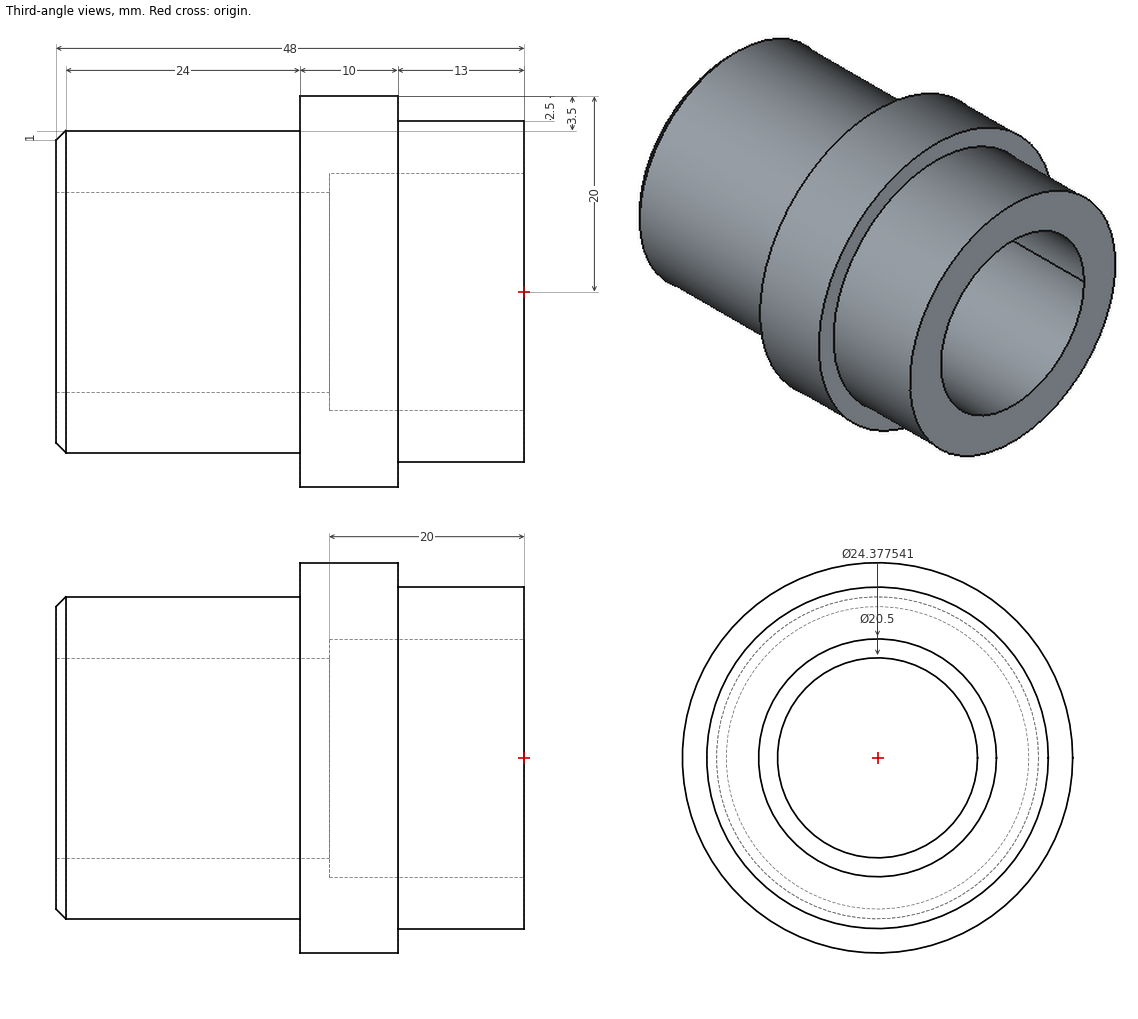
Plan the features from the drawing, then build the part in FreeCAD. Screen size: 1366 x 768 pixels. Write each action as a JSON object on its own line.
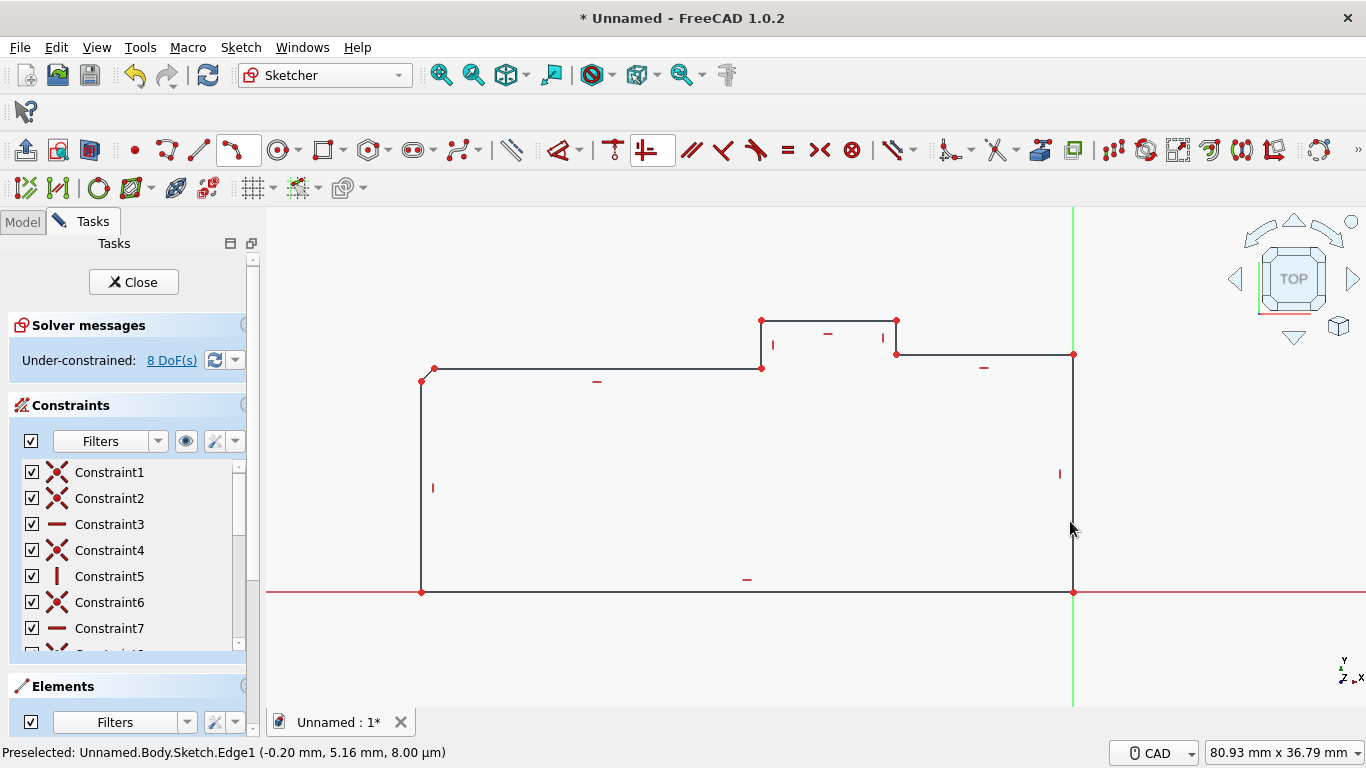
{"action": "left_click", "coordinate": [558, 150]}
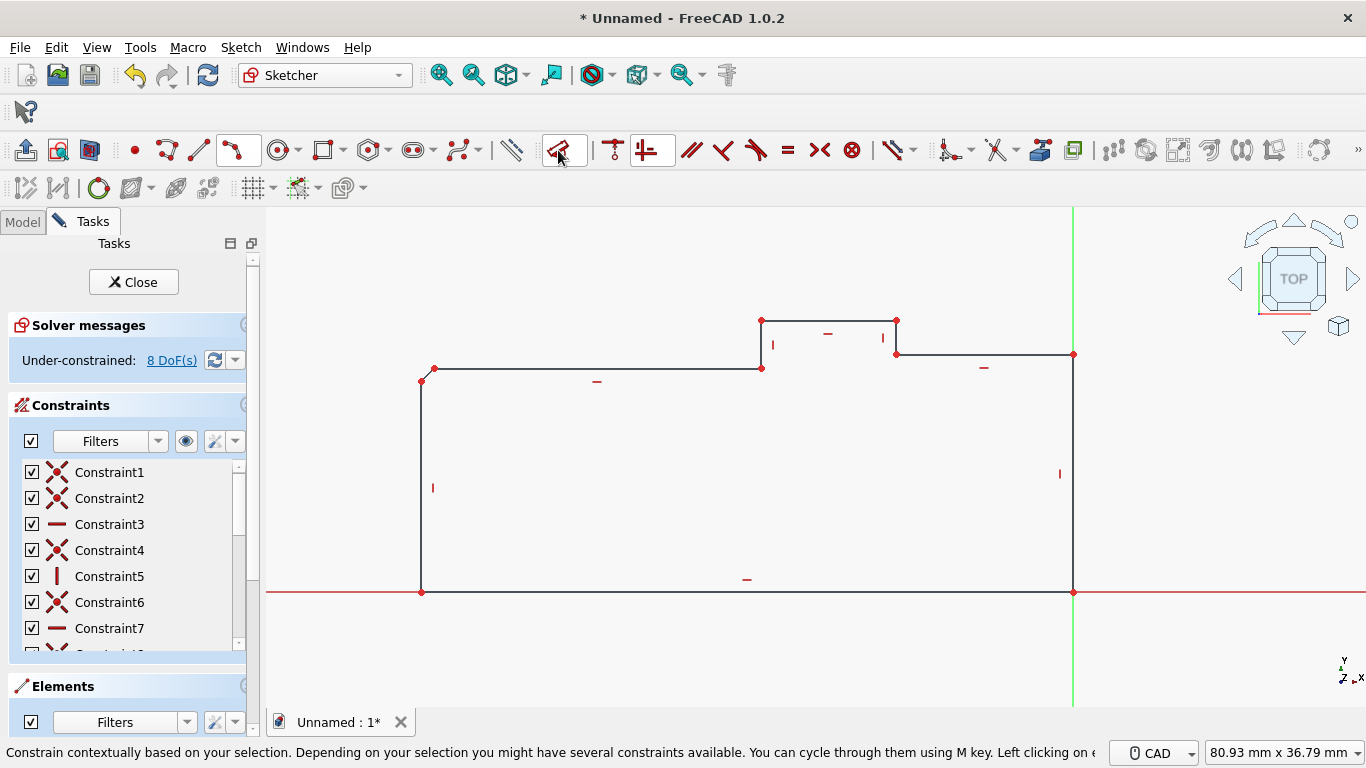
{"action": "left_click", "coordinate": [1020, 355]}
{"action": "left_click", "coordinate": [985, 321]}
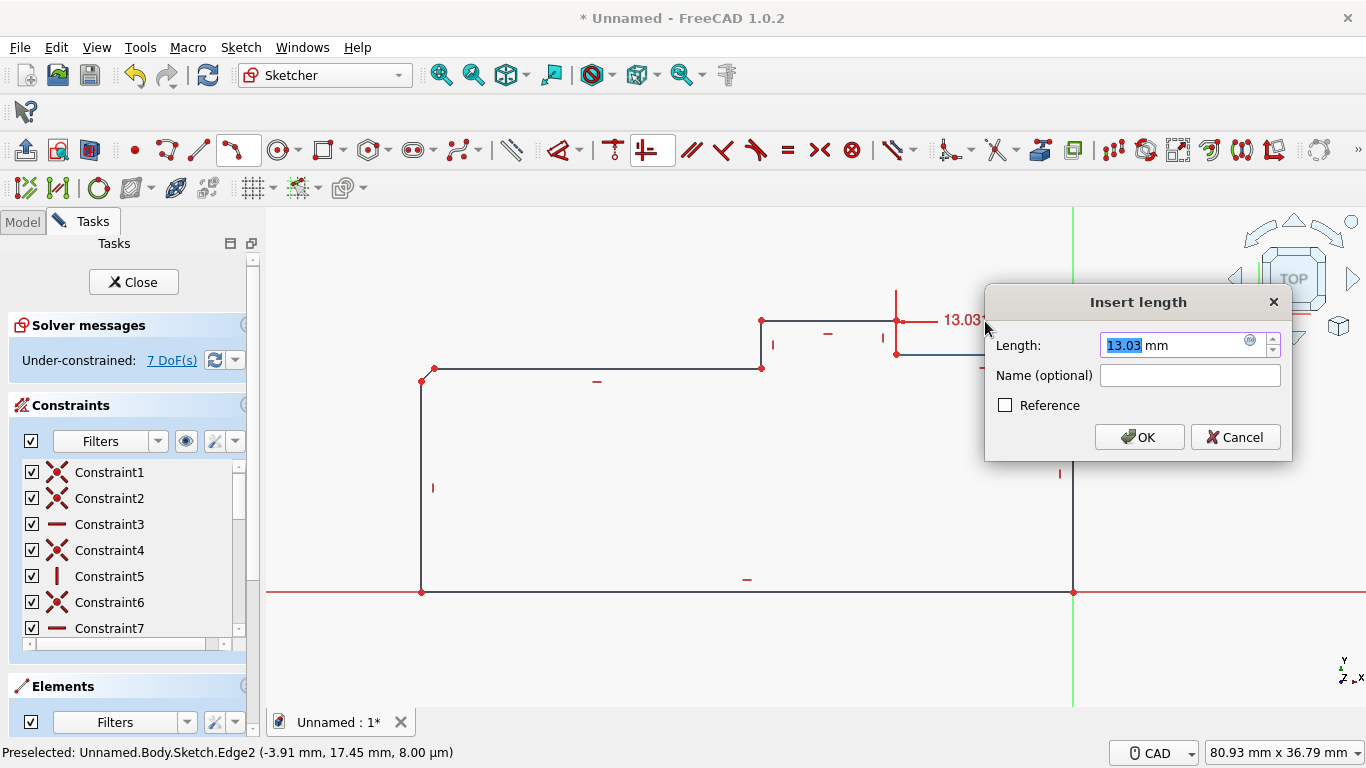
{"action": "type", "text": "13"}
{"action": "key", "text": "Return"}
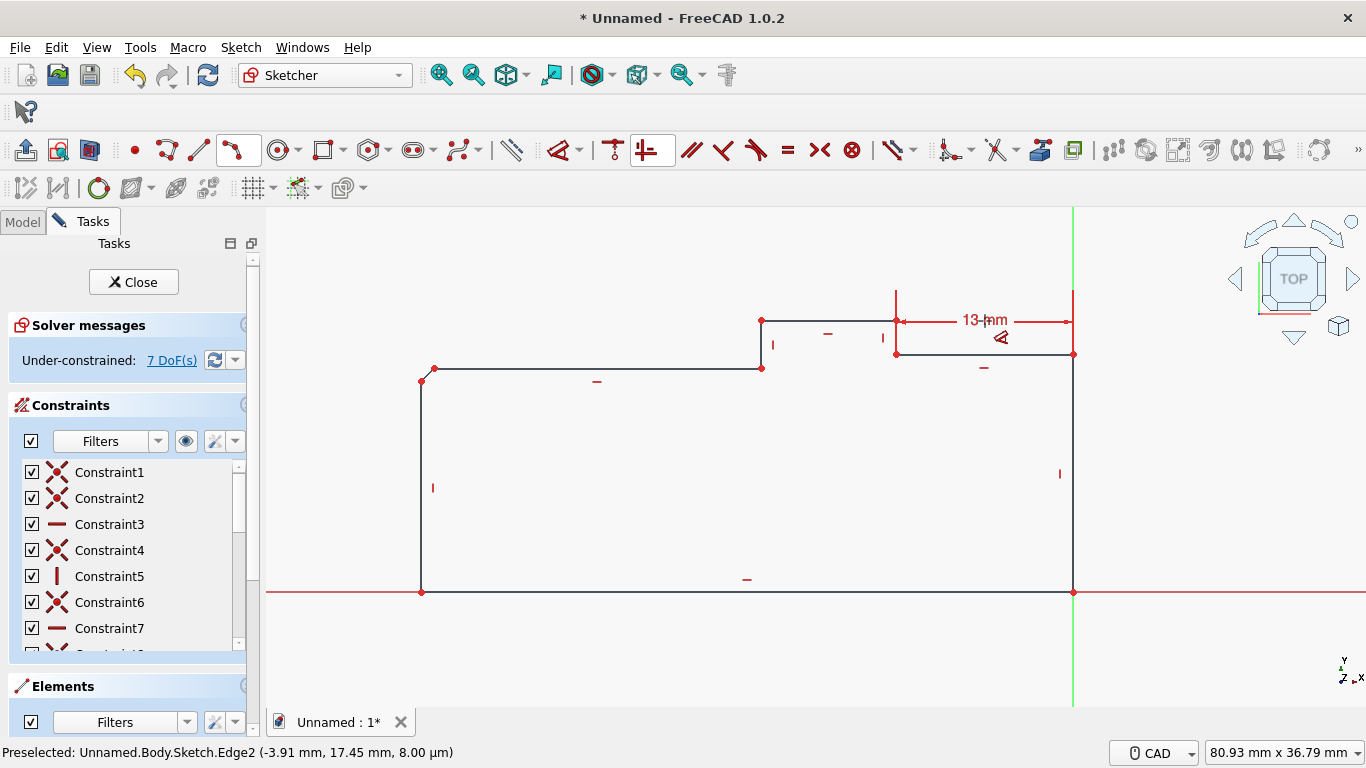
{"action": "left_click", "coordinate": [856, 321]}
{"action": "left_click", "coordinate": [829, 287]}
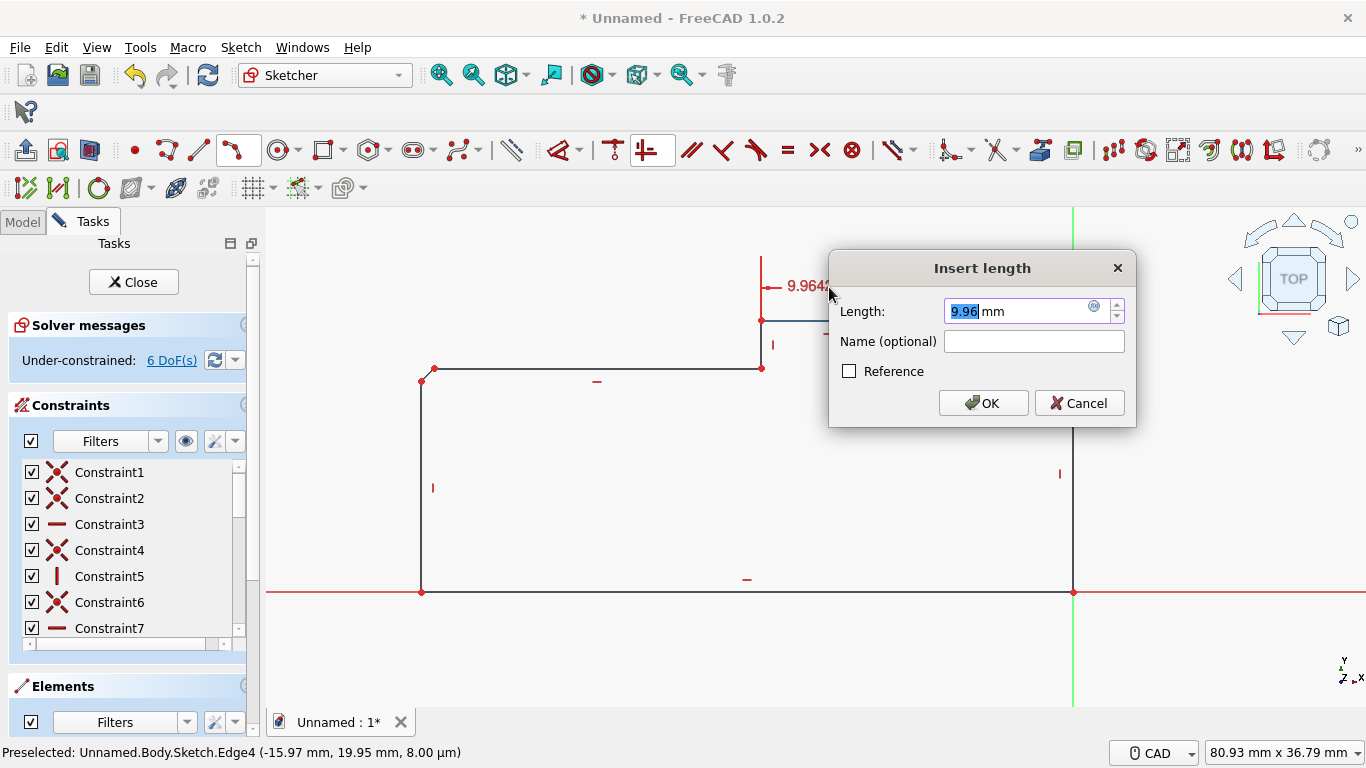
{"action": "type", "text": "10"}
{"action": "key", "text": "Return"}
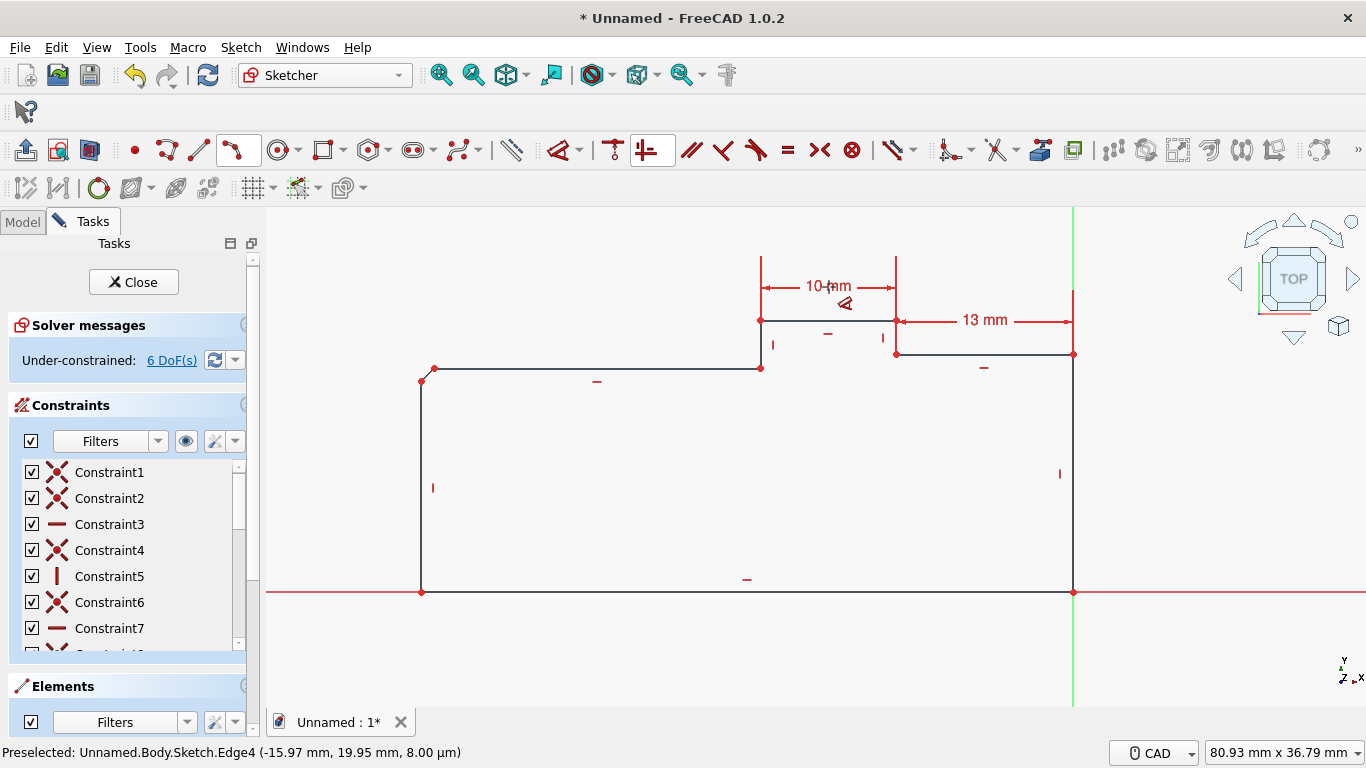
{"action": "left_click", "coordinate": [663, 369]}
{"action": "left_click", "coordinate": [597, 335]}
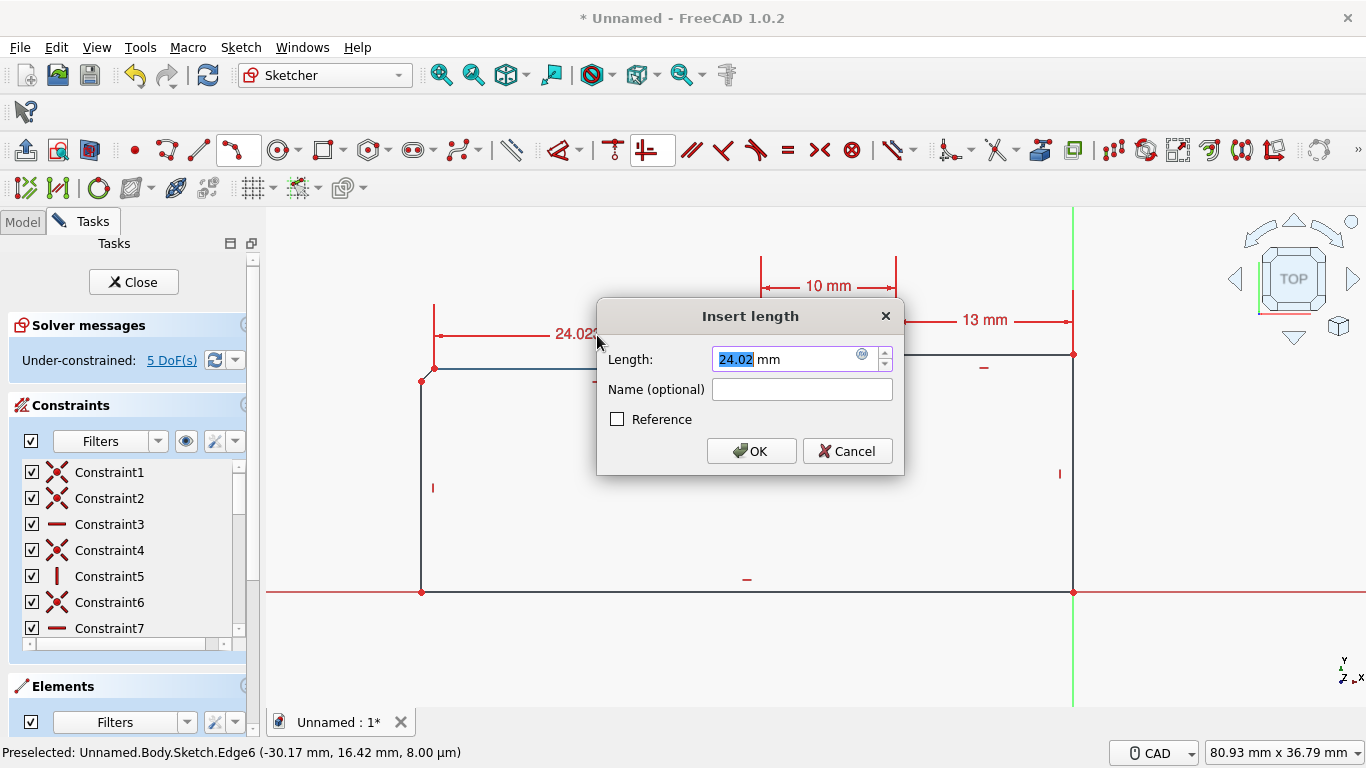
{"action": "type", "text": "24"}
{"action": "key", "text": "Return"}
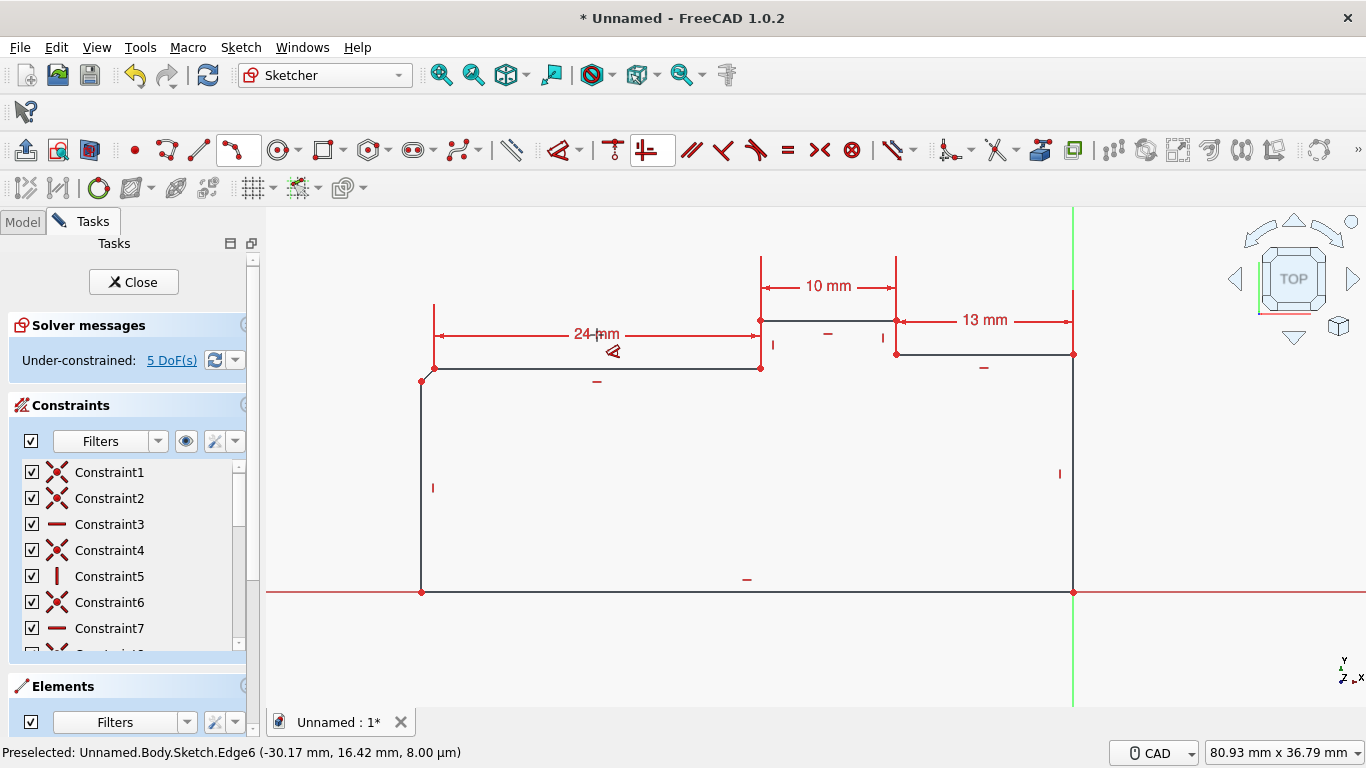
{"action": "left_click", "coordinate": [617, 592]}
{"action": "left_click", "coordinate": [747, 626]}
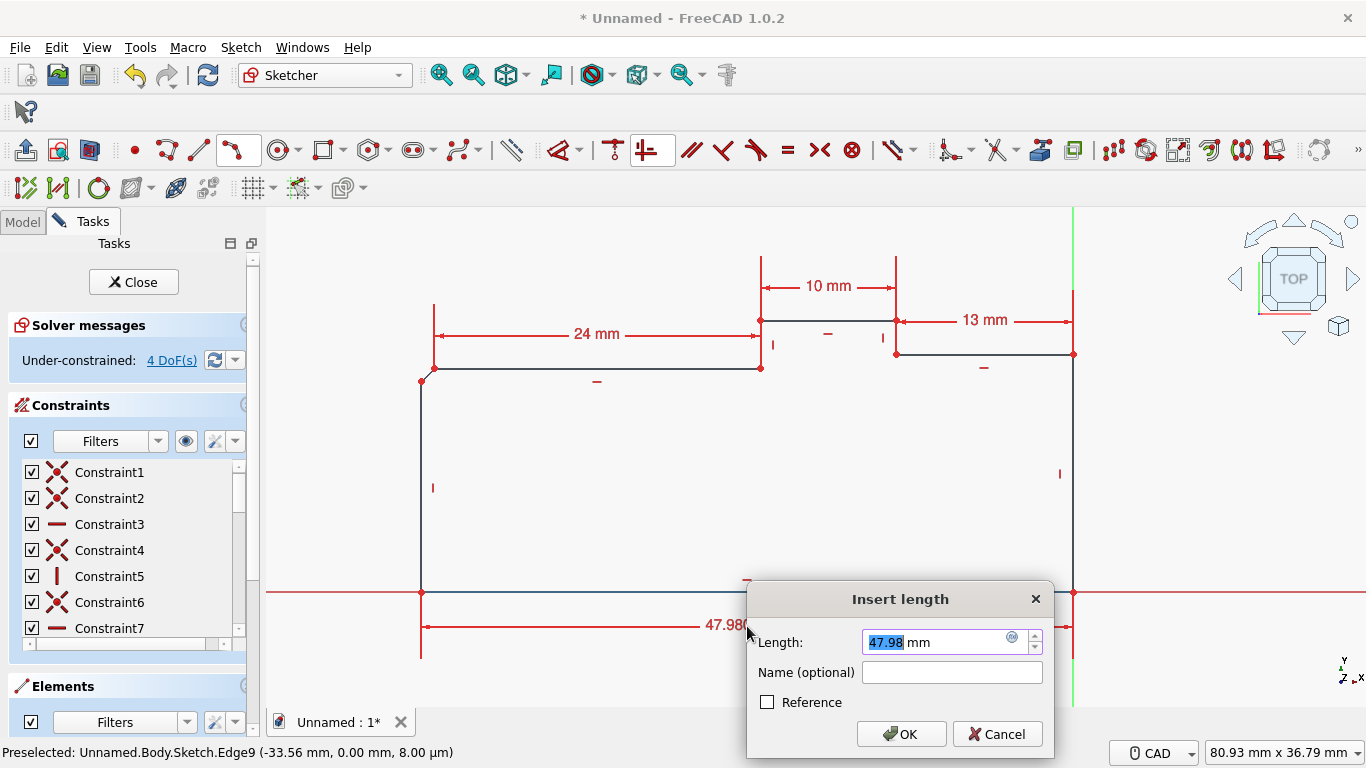
{"action": "type", "text": "48"}
{"action": "key", "text": "Return"}